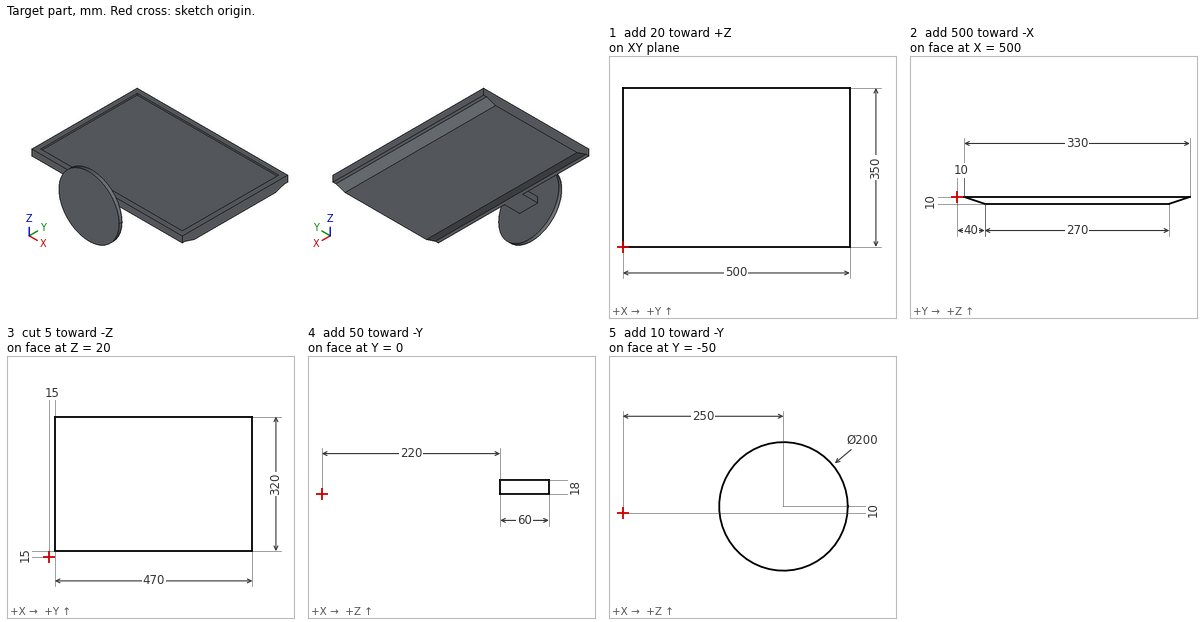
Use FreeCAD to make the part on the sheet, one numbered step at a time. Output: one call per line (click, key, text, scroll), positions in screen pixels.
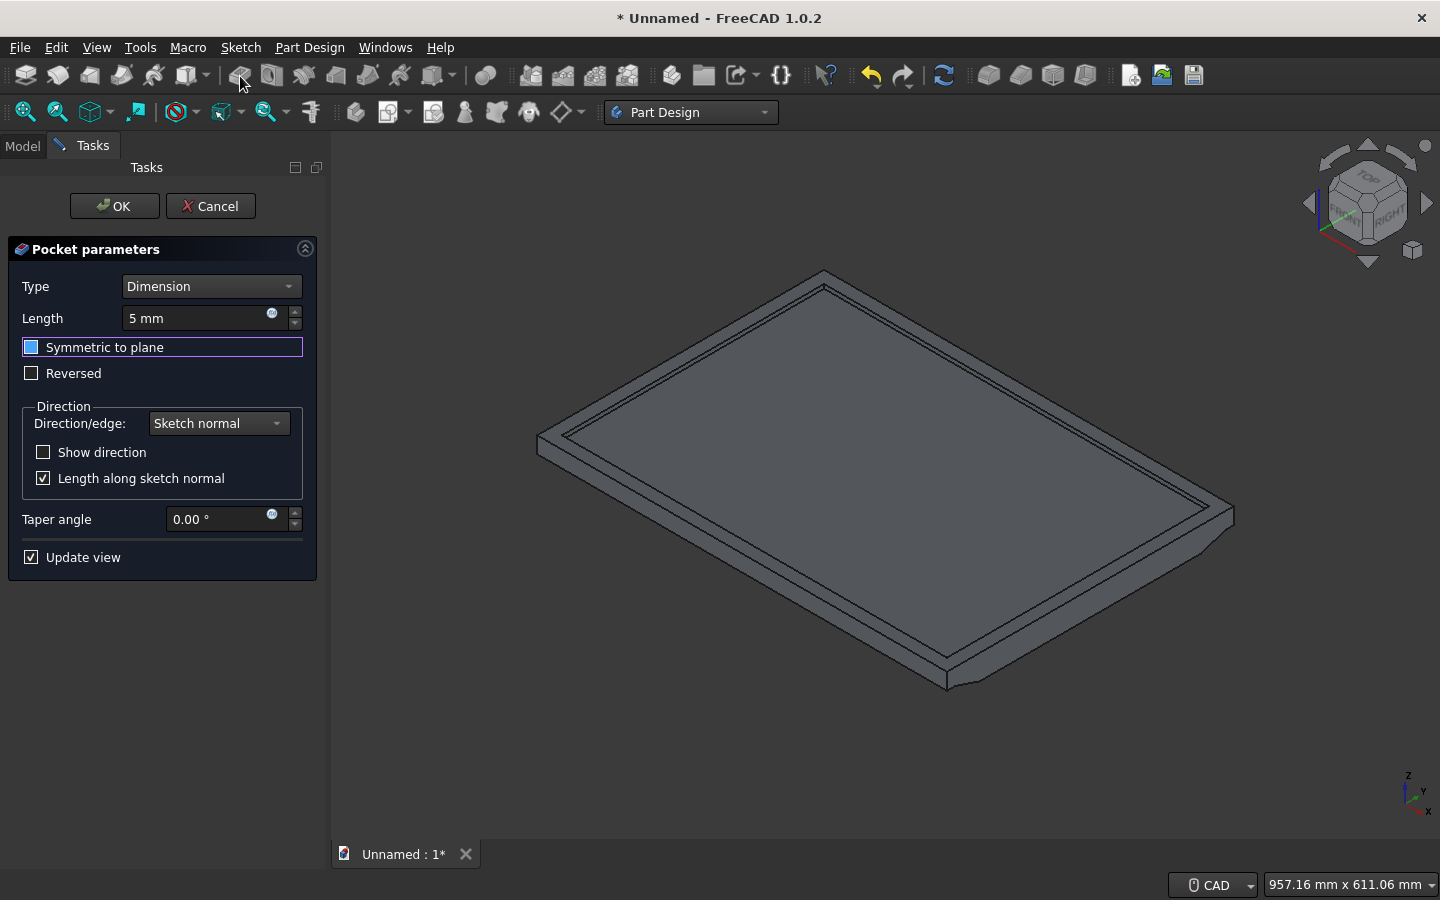
click(115, 206)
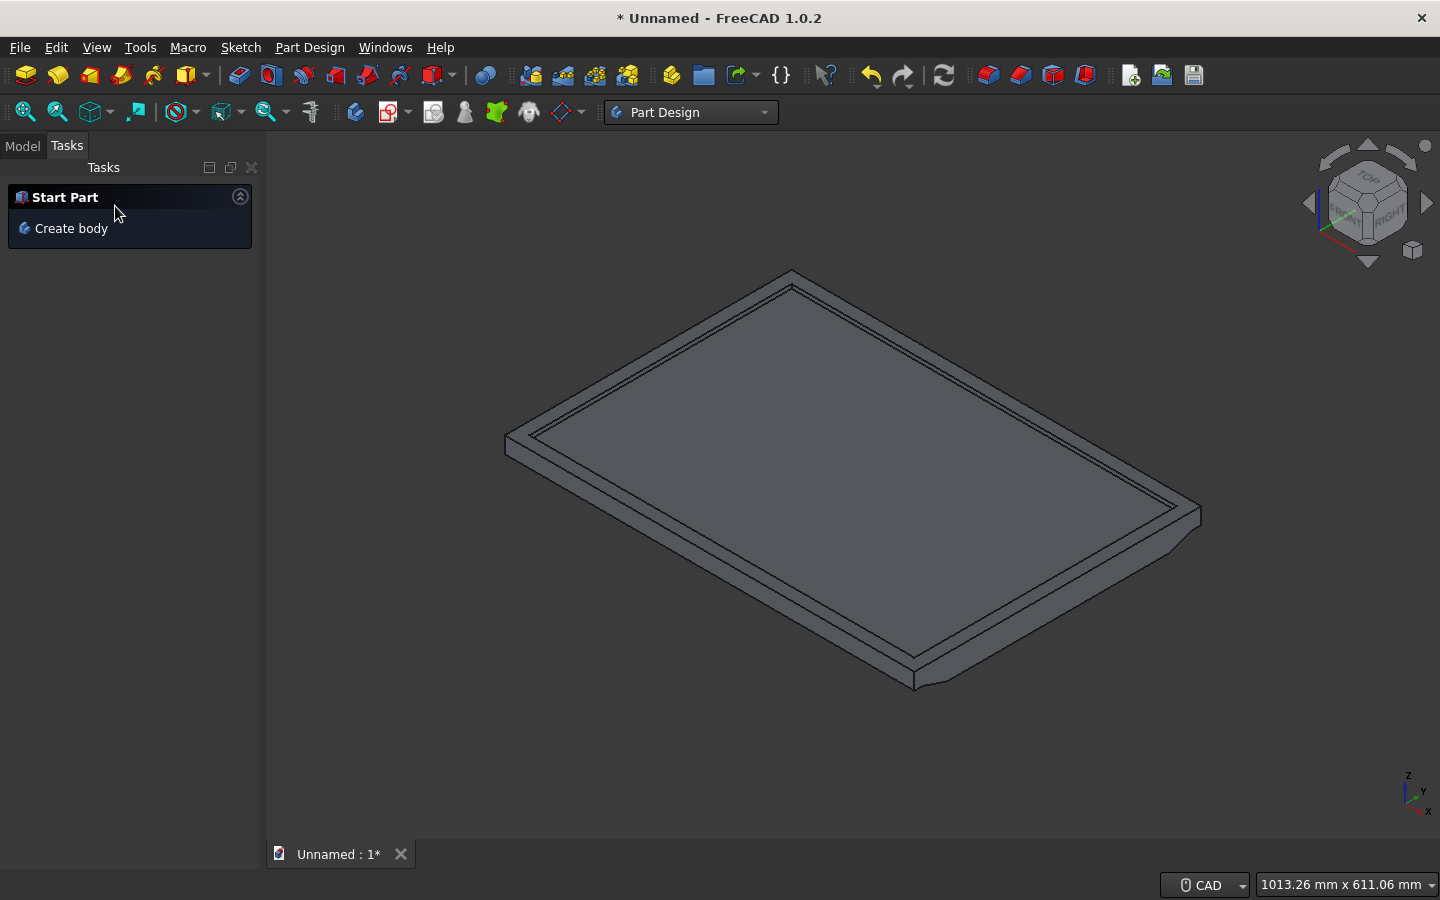
key(1)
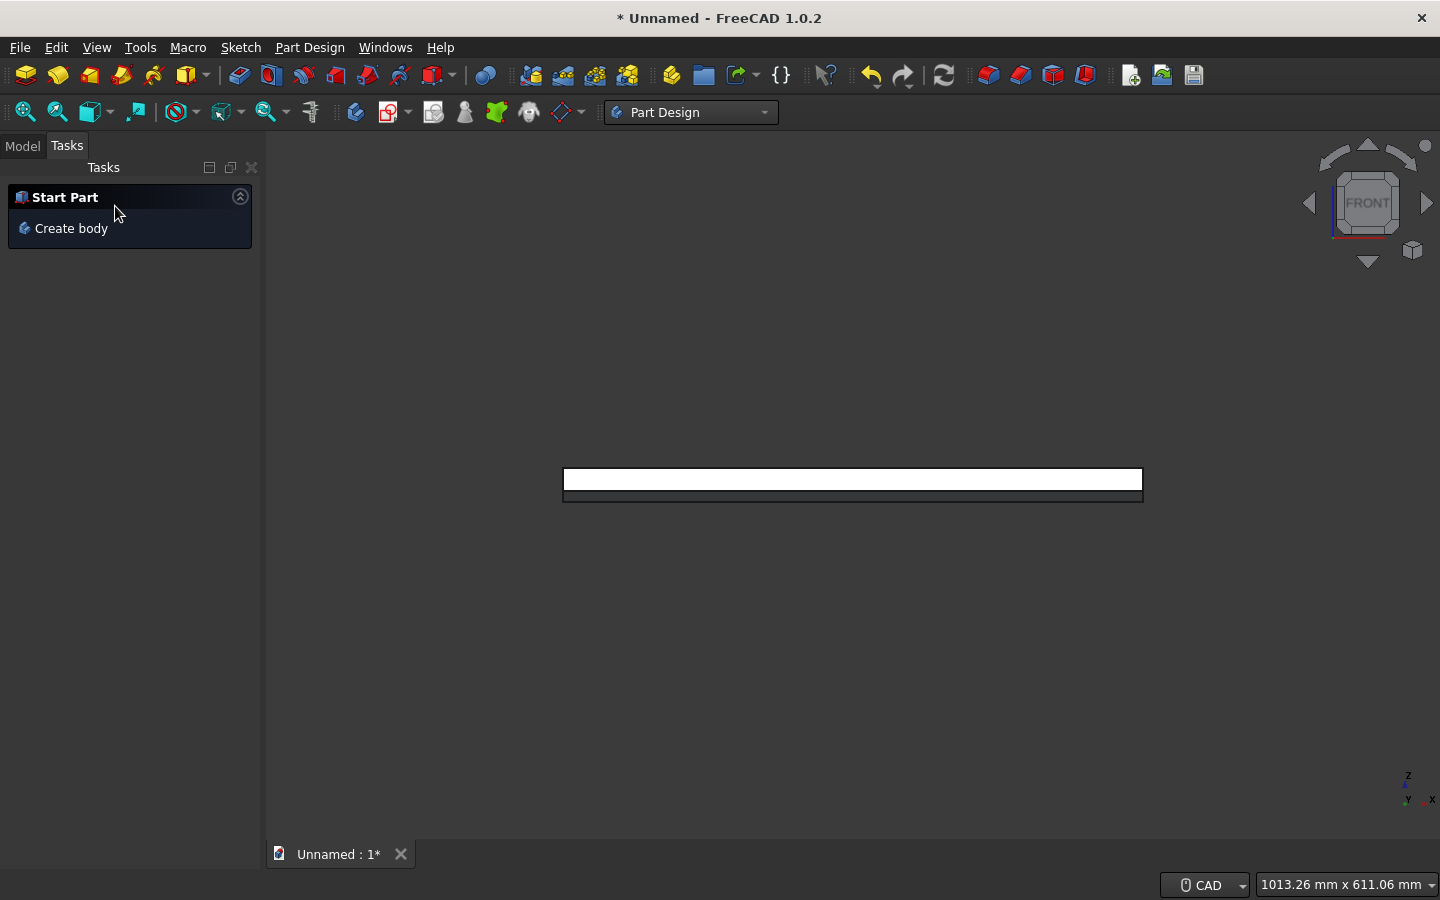
click(1101, 478)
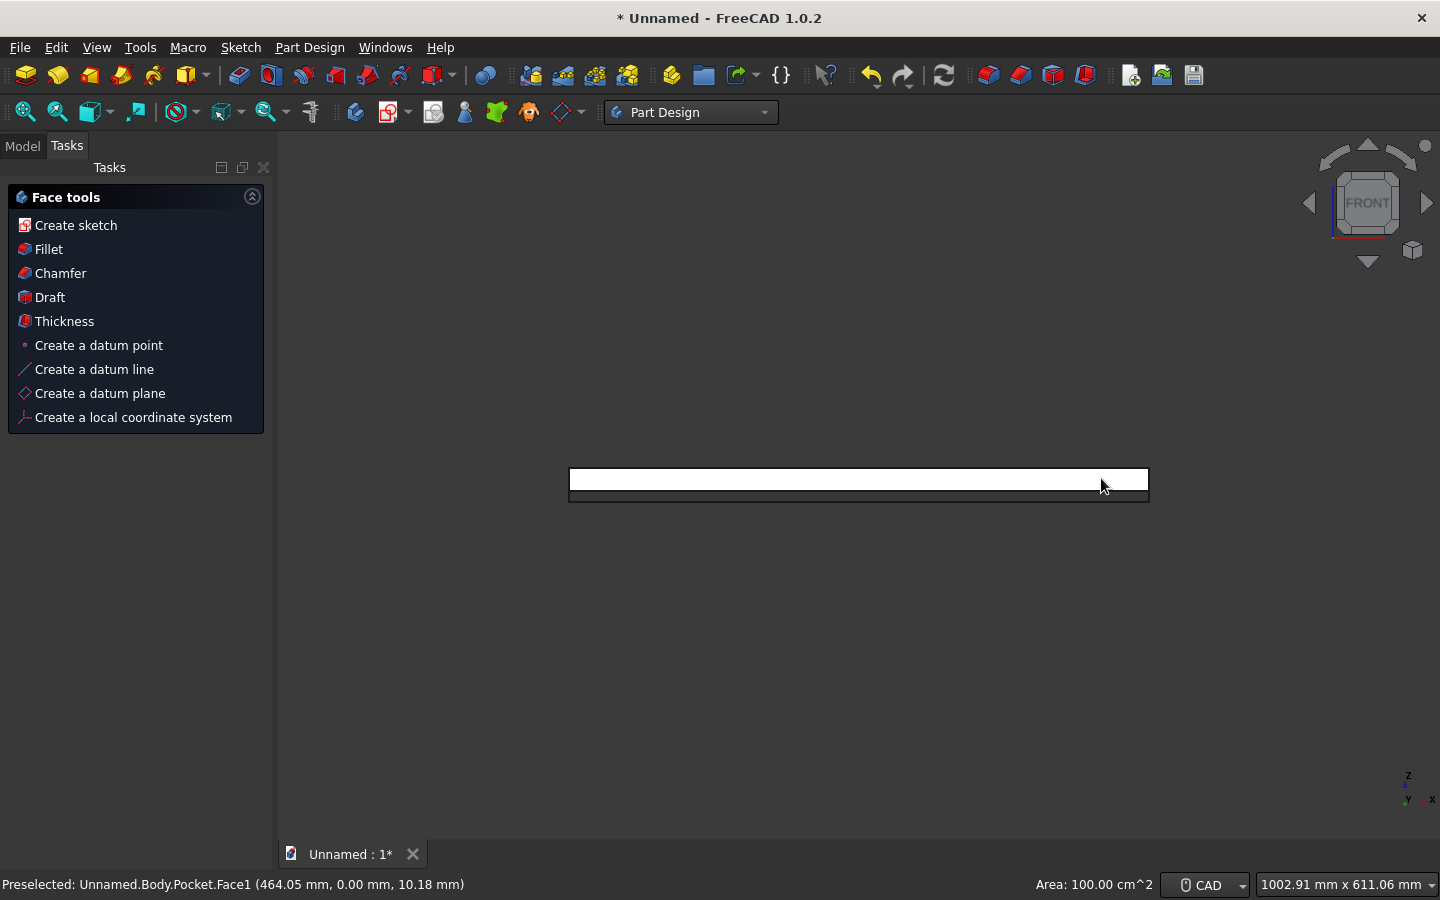
click(388, 112)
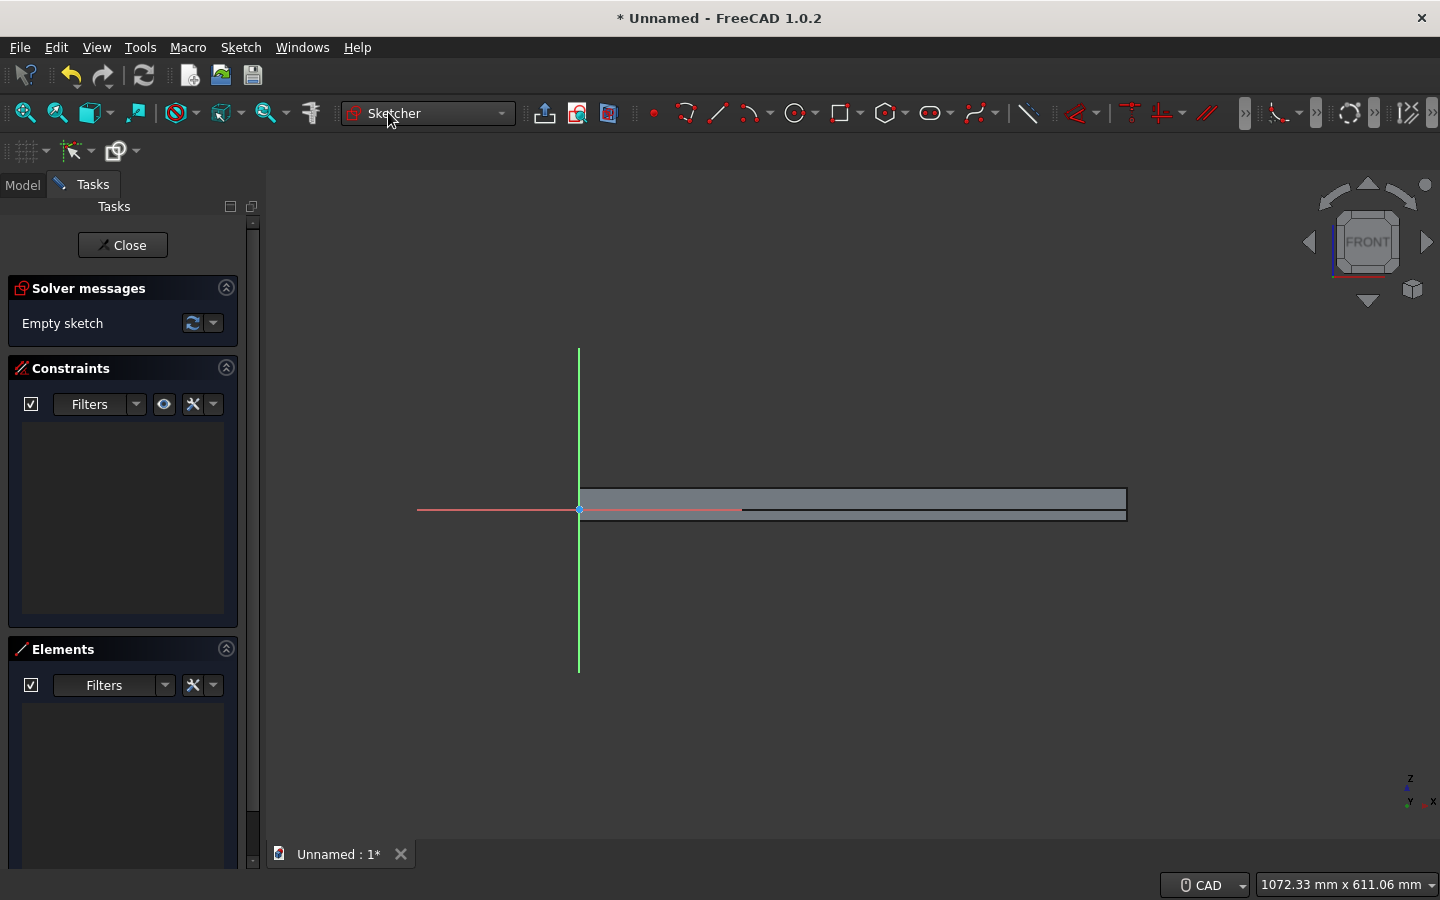
scroll(860, 500, up, 12)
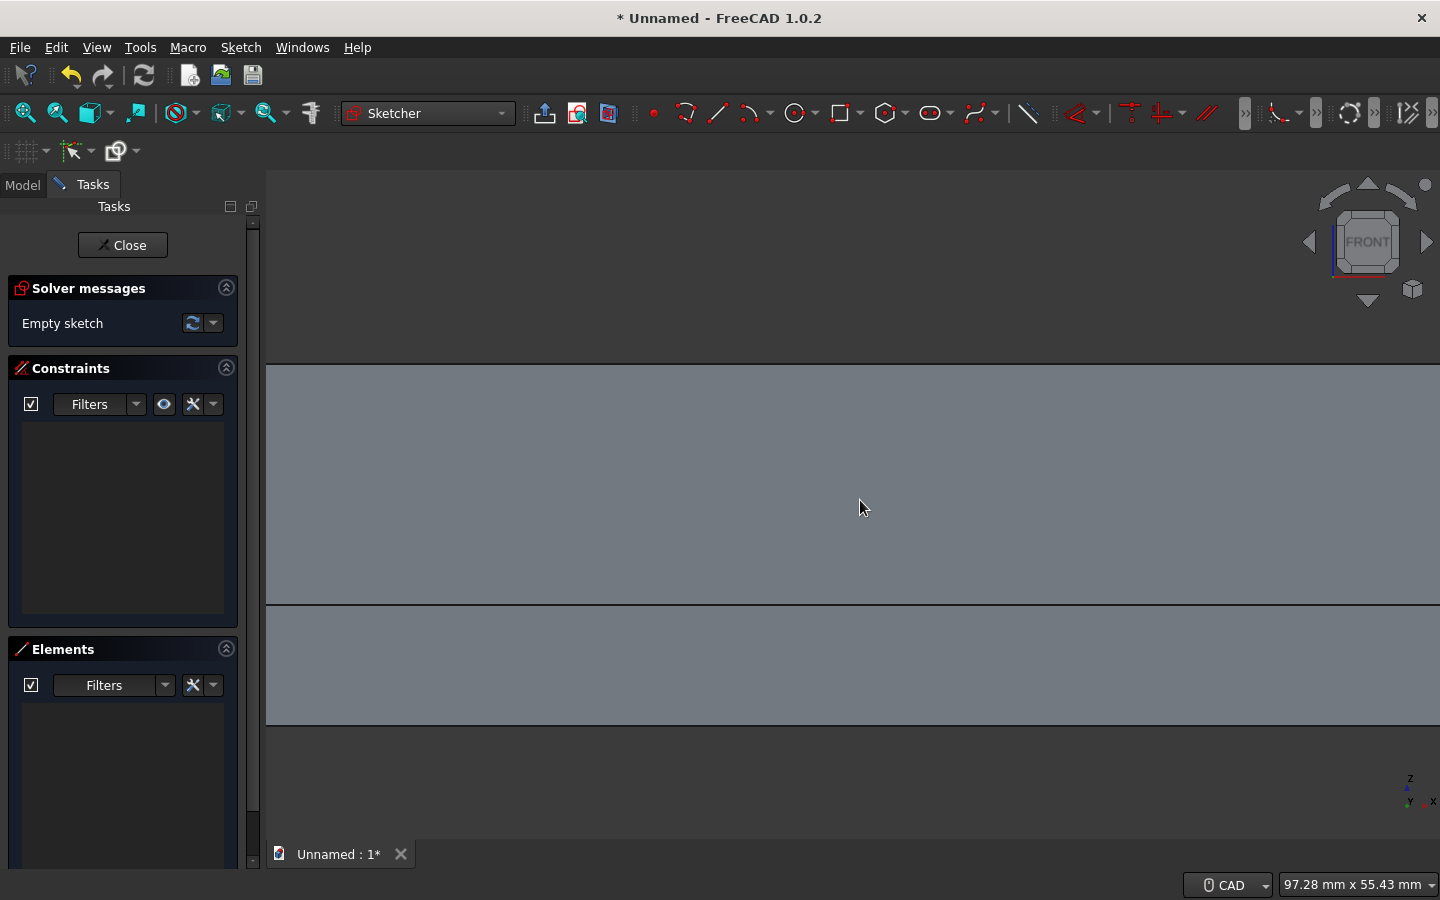
click(840, 114)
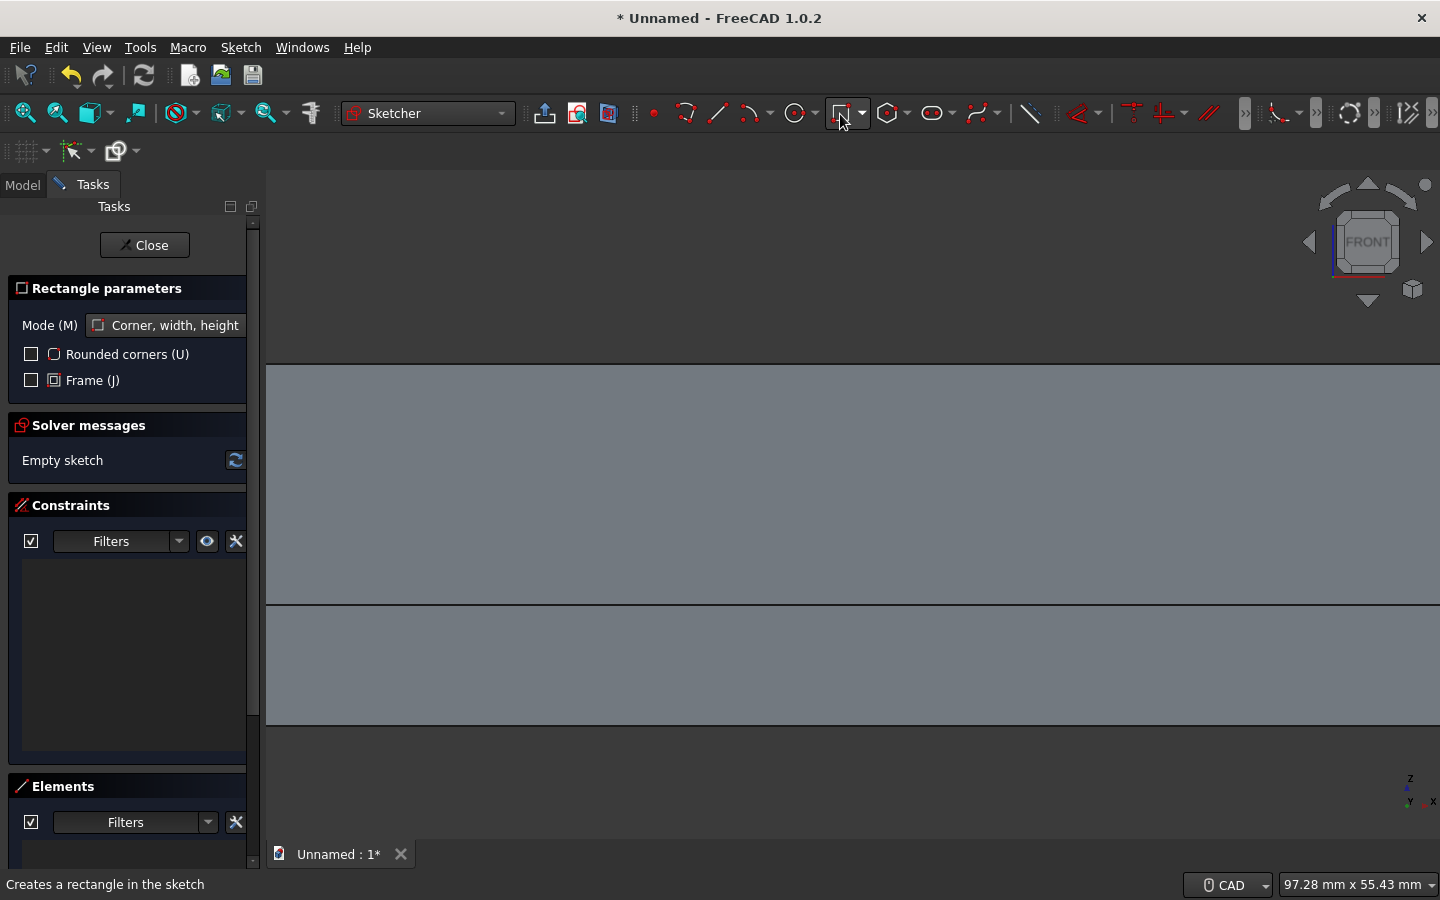
click(416, 388)
click(1140, 605)
key(Escape)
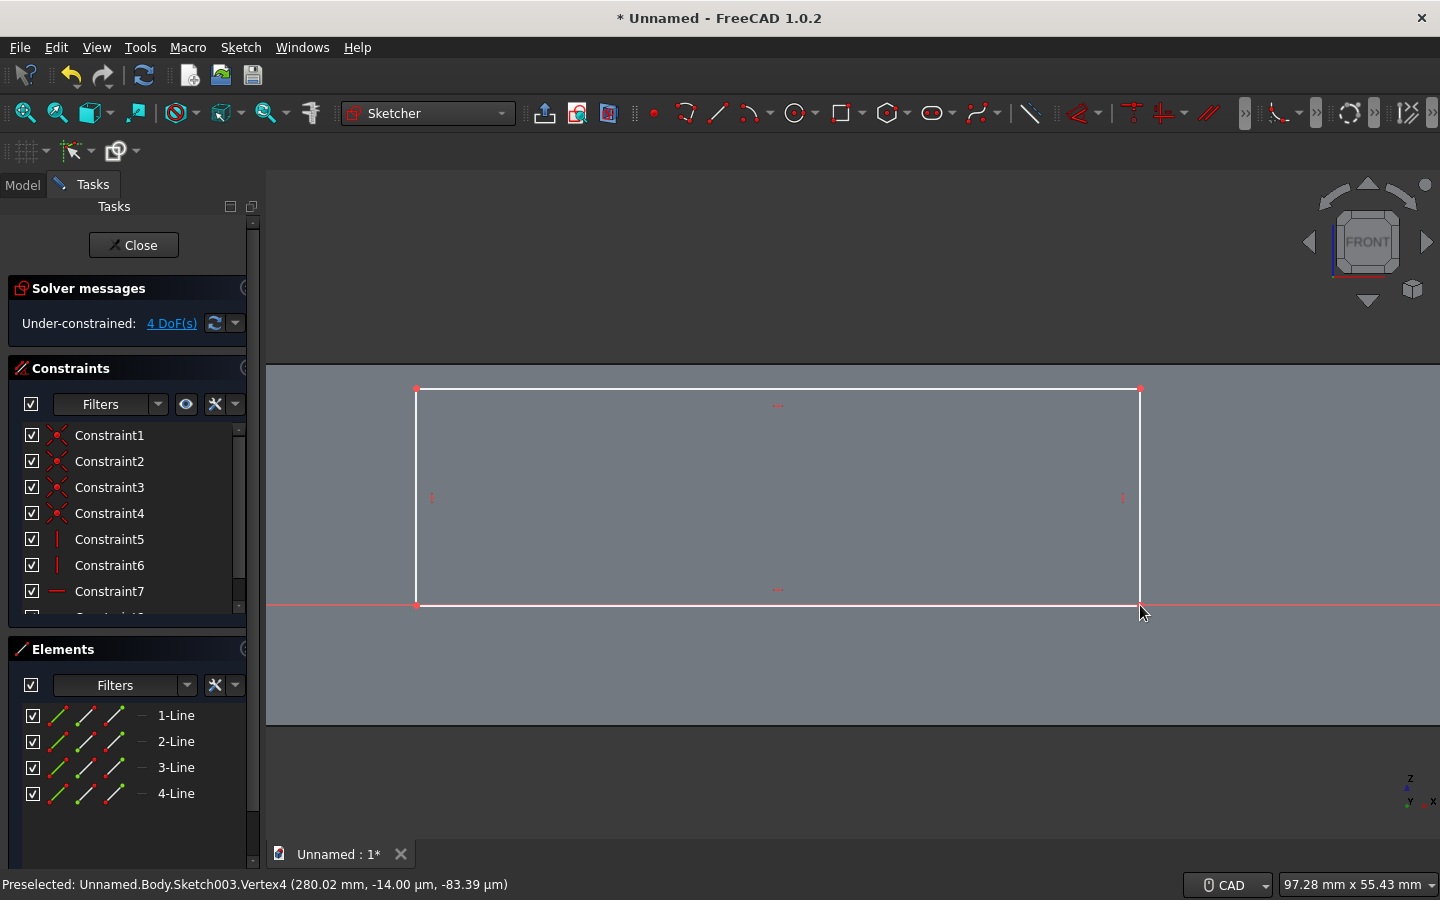
click(416, 606)